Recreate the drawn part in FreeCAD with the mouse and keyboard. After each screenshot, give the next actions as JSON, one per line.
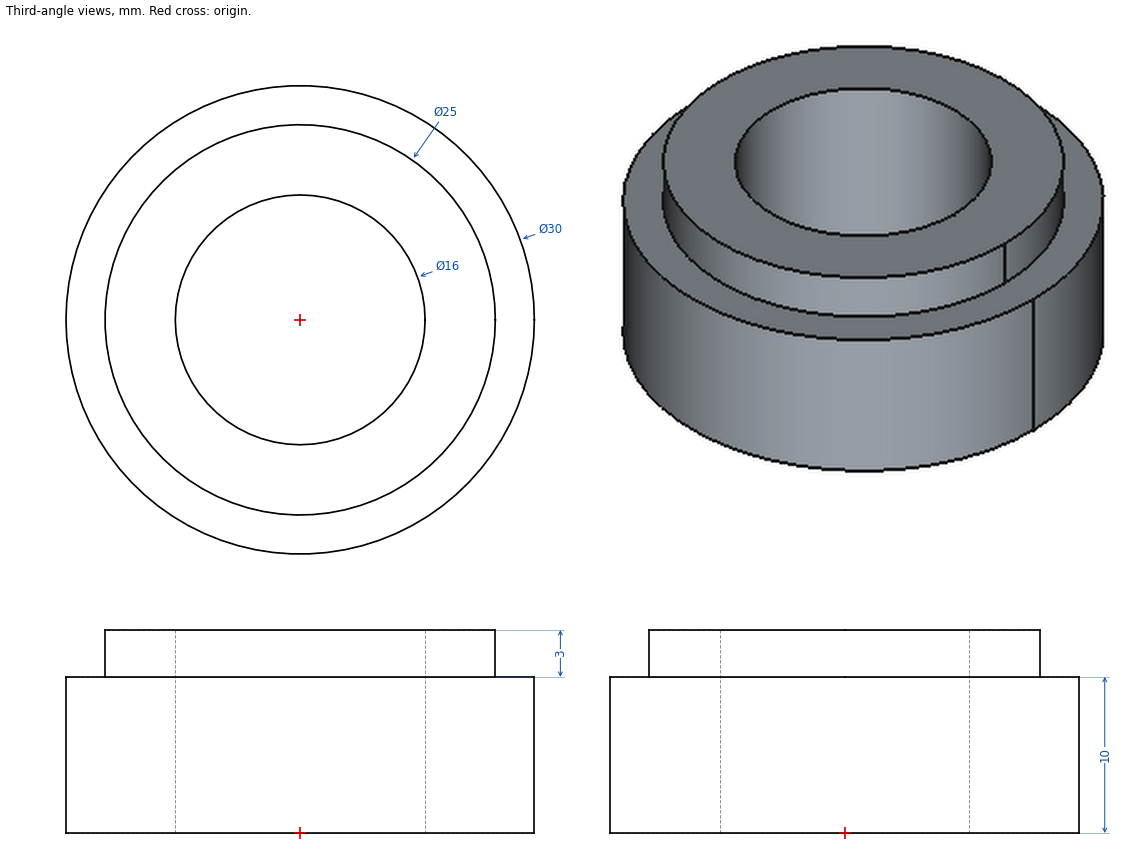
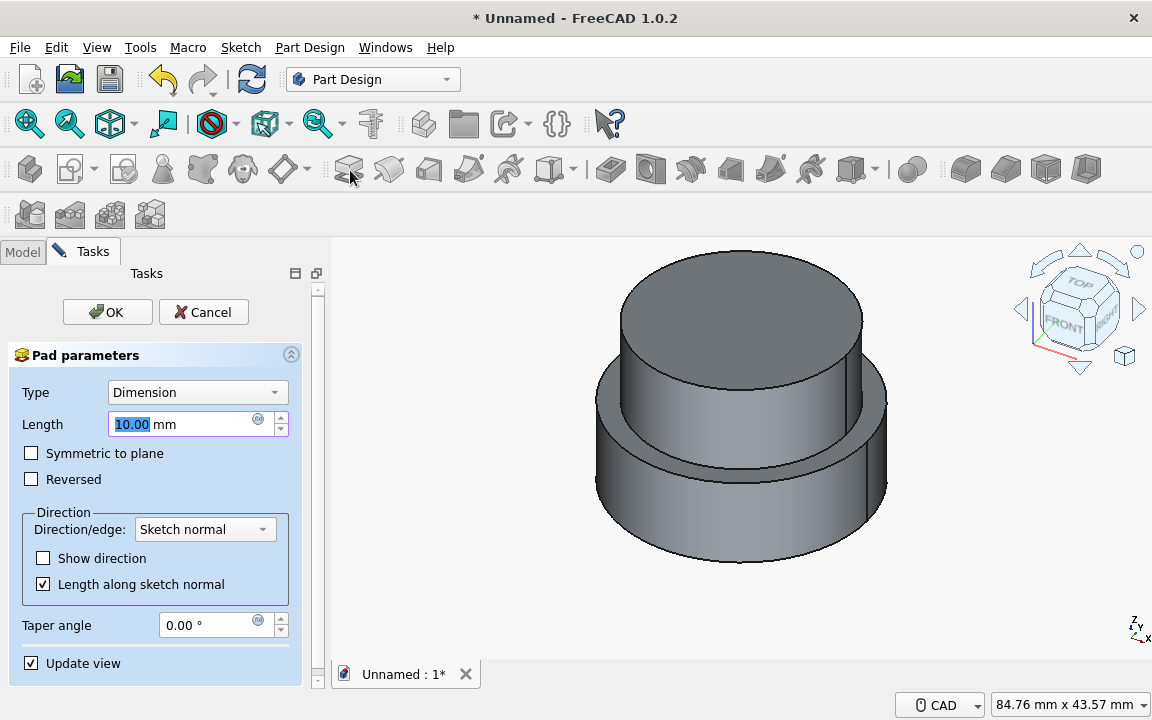
{"action": "type", "text": "3"}
{"action": "key", "text": "Tab"}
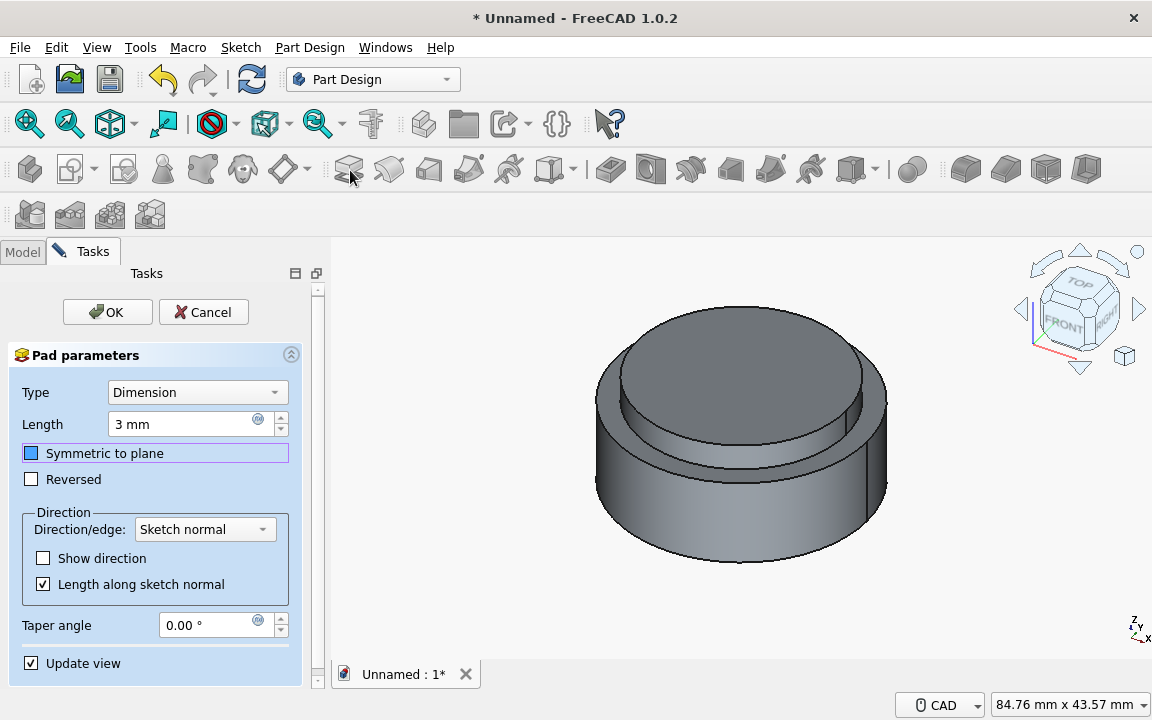
{"action": "left_click", "coordinate": [108, 312]}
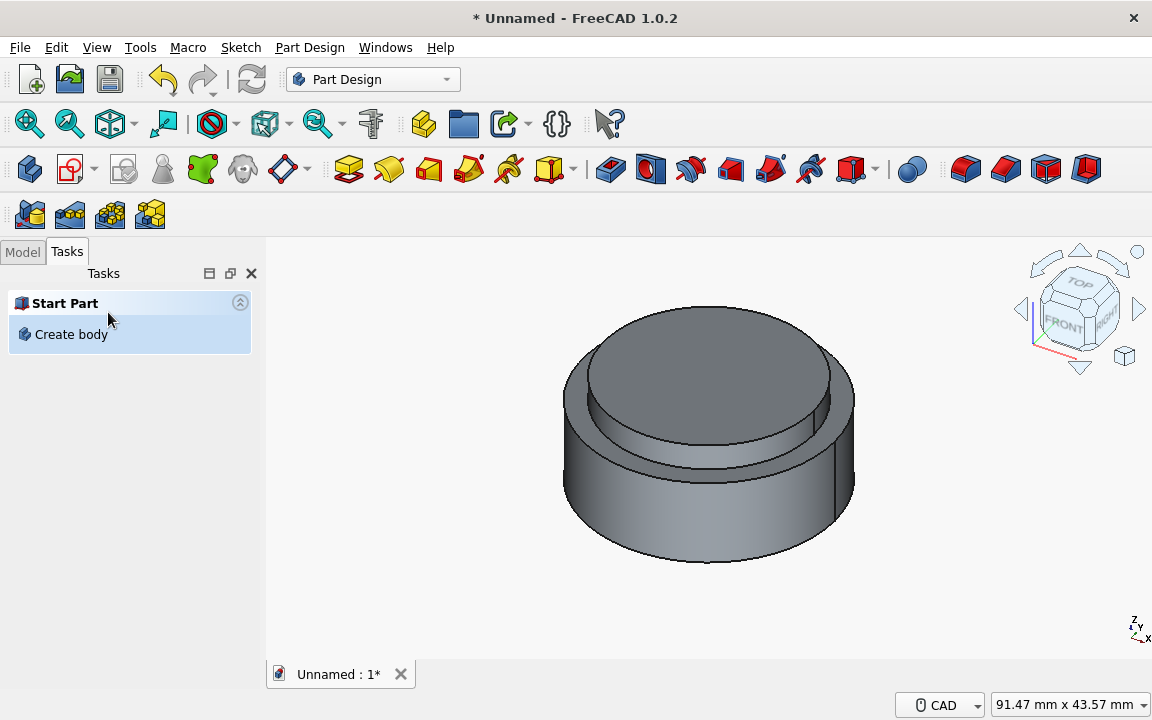
{"action": "left_click", "coordinate": [709, 375]}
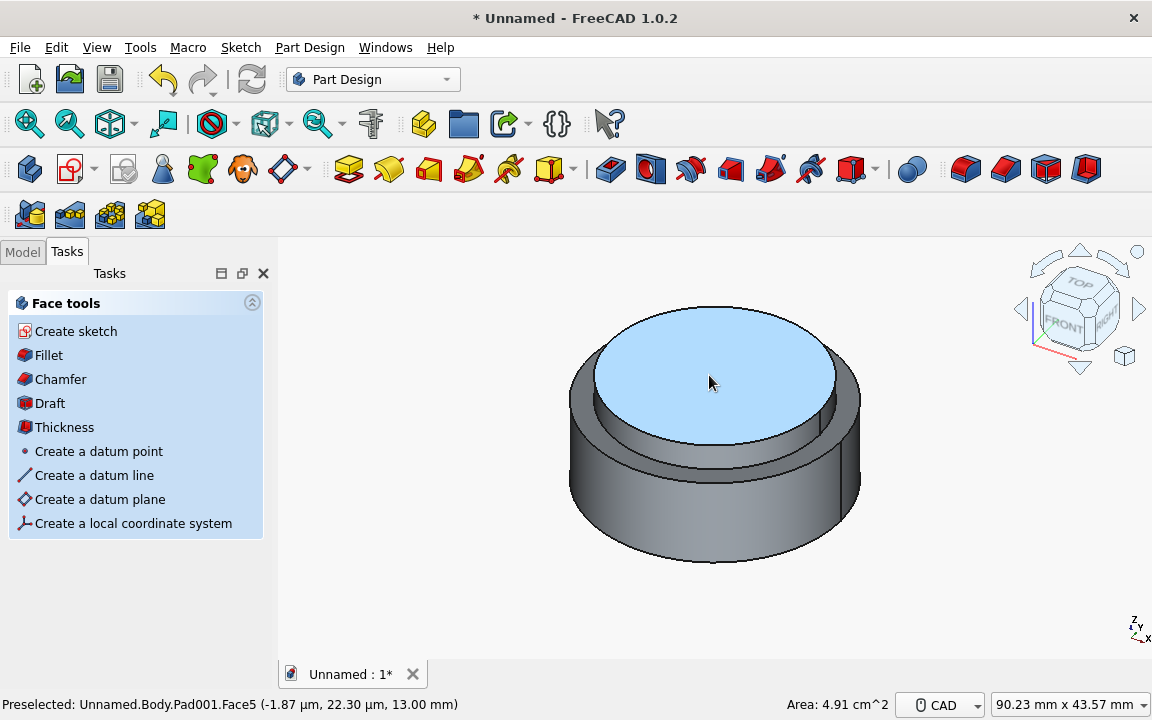
{"action": "left_click", "coordinate": [70, 170]}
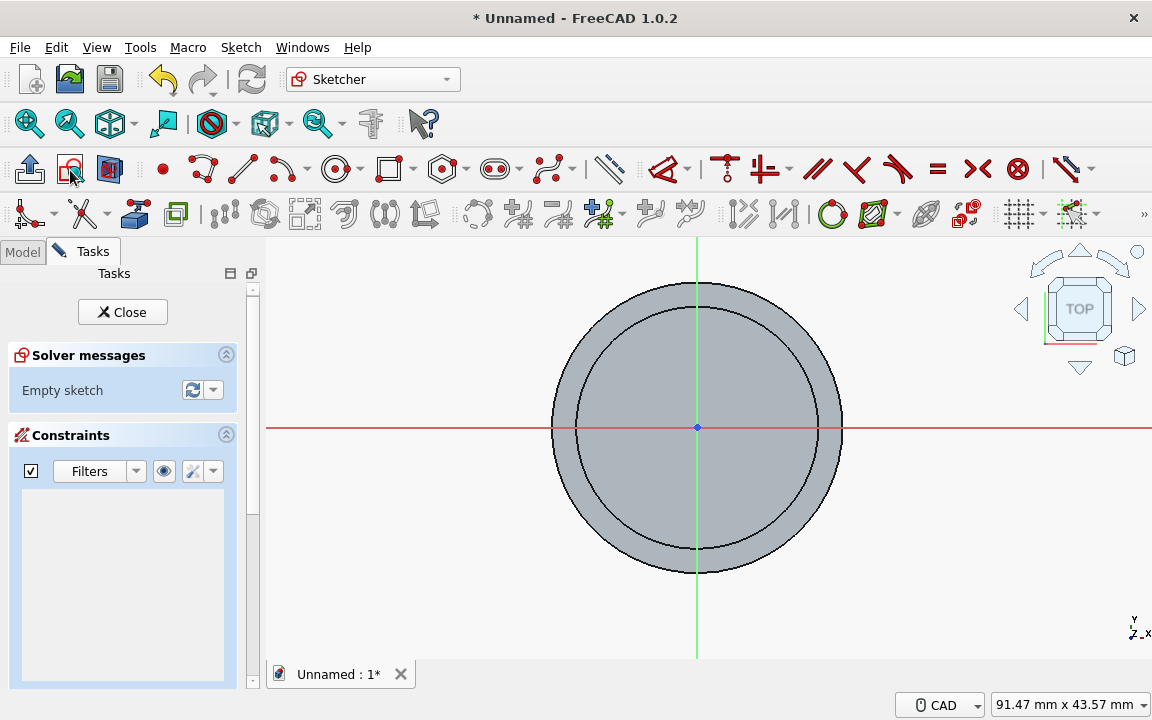
{"action": "scroll", "coordinate": [766, 403], "scroll_direction": "up", "scroll_amount": 3}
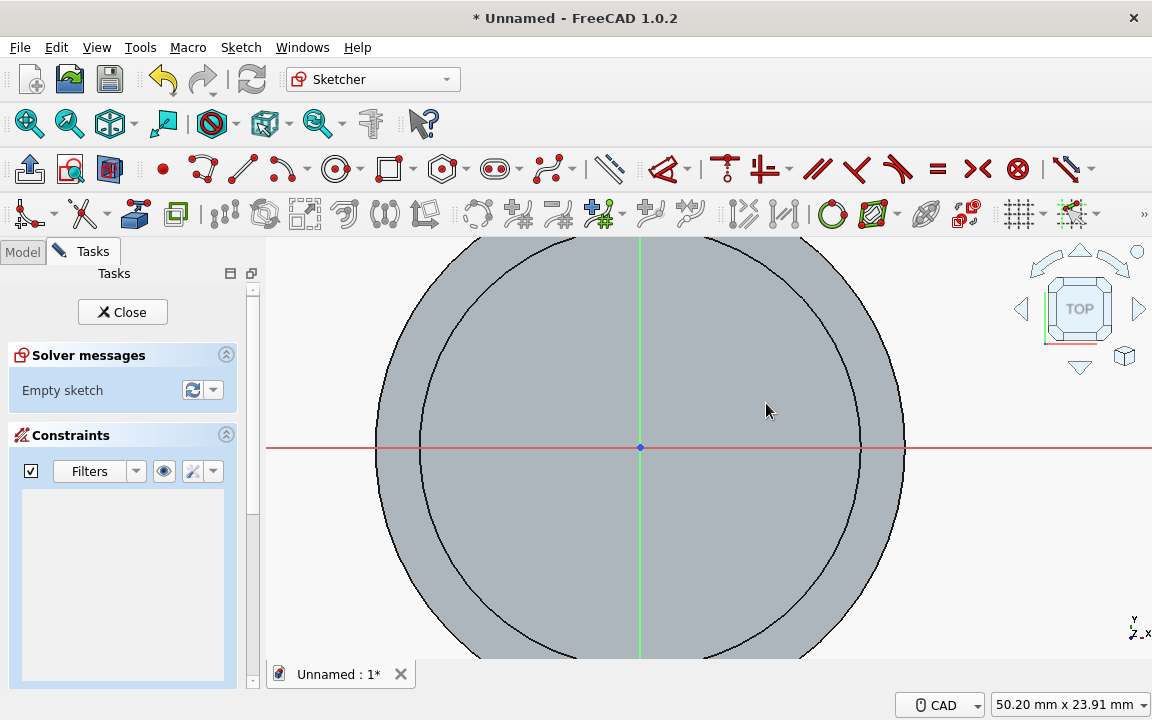
{"action": "key", "text": "g c"}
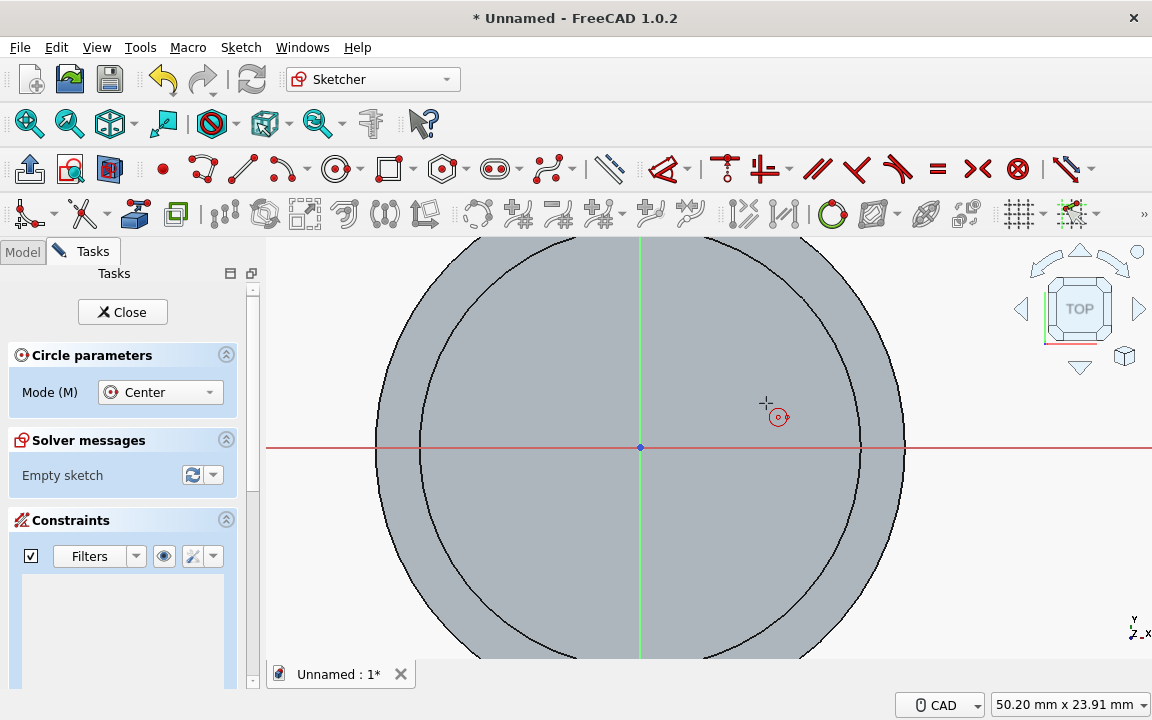
{"action": "left_click", "coordinate": [640, 448]}
{"action": "left_click", "coordinate": [740, 348]}
{"action": "key", "text": "Escape"}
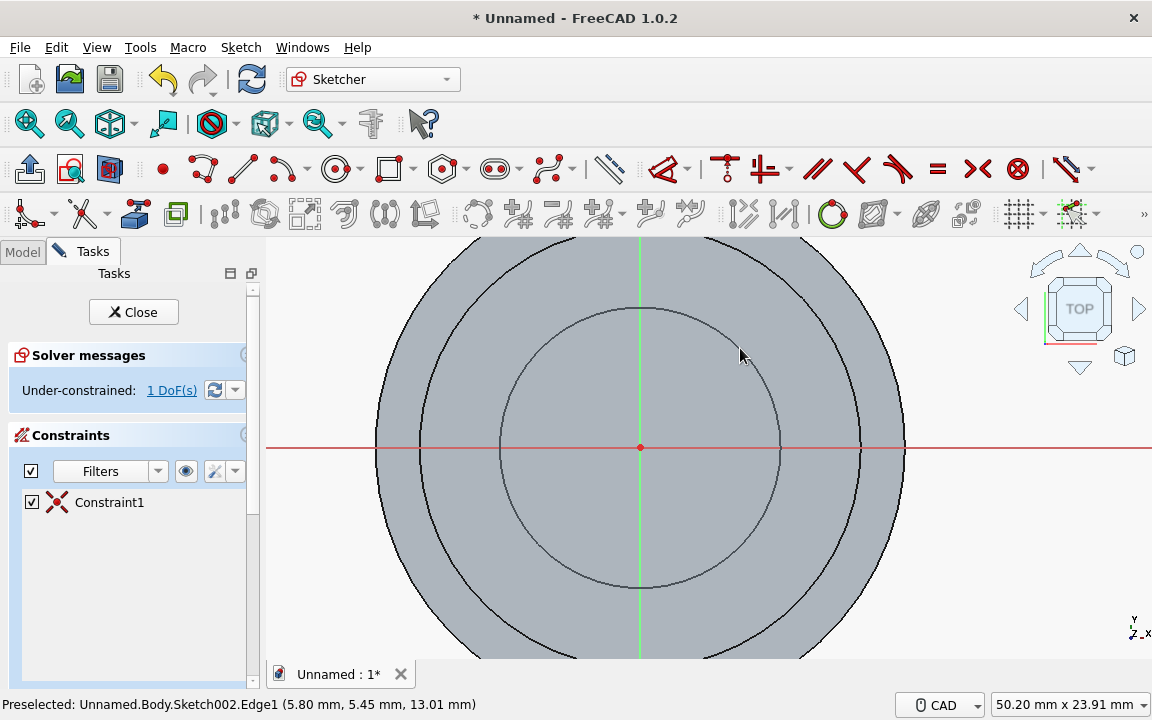
{"action": "left_click", "coordinate": [739, 348]}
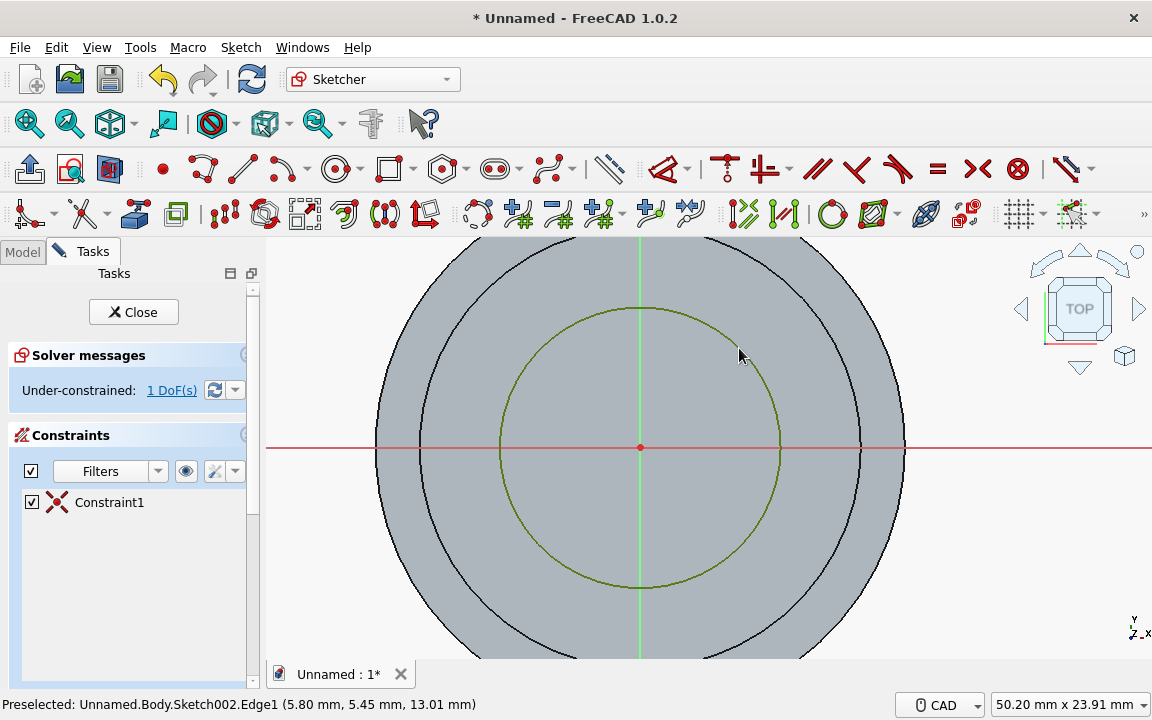
{"action": "left_click", "coordinate": [690, 170]}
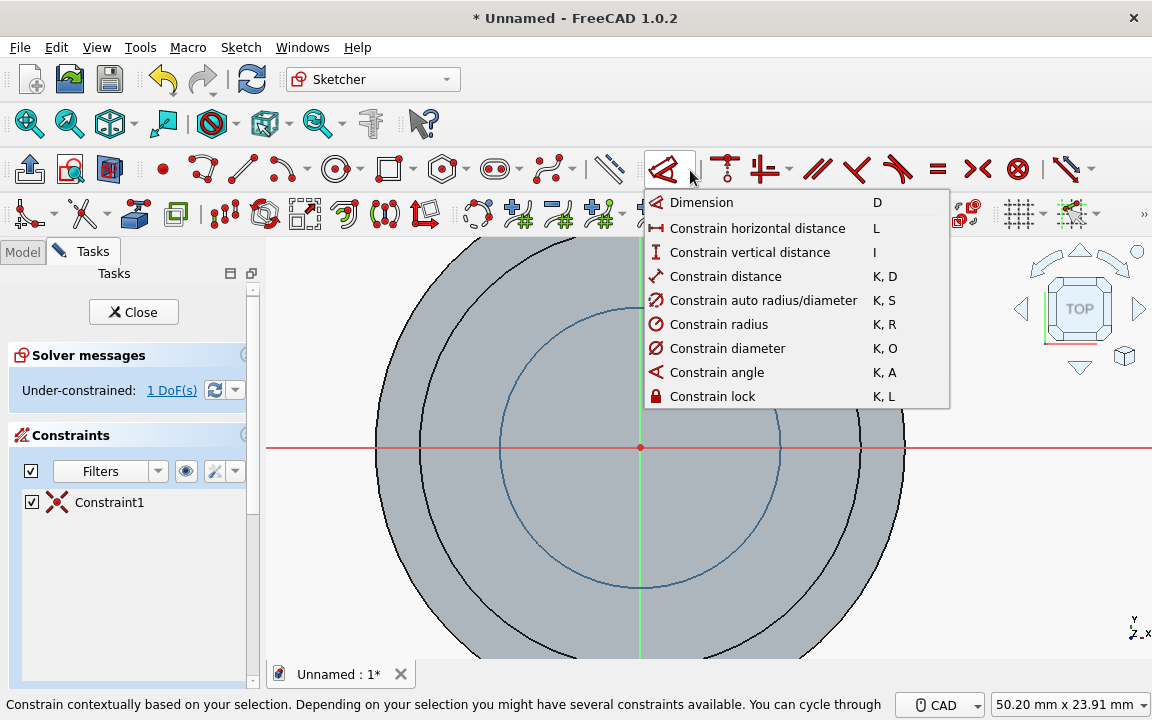
{"action": "left_click", "coordinate": [797, 348]}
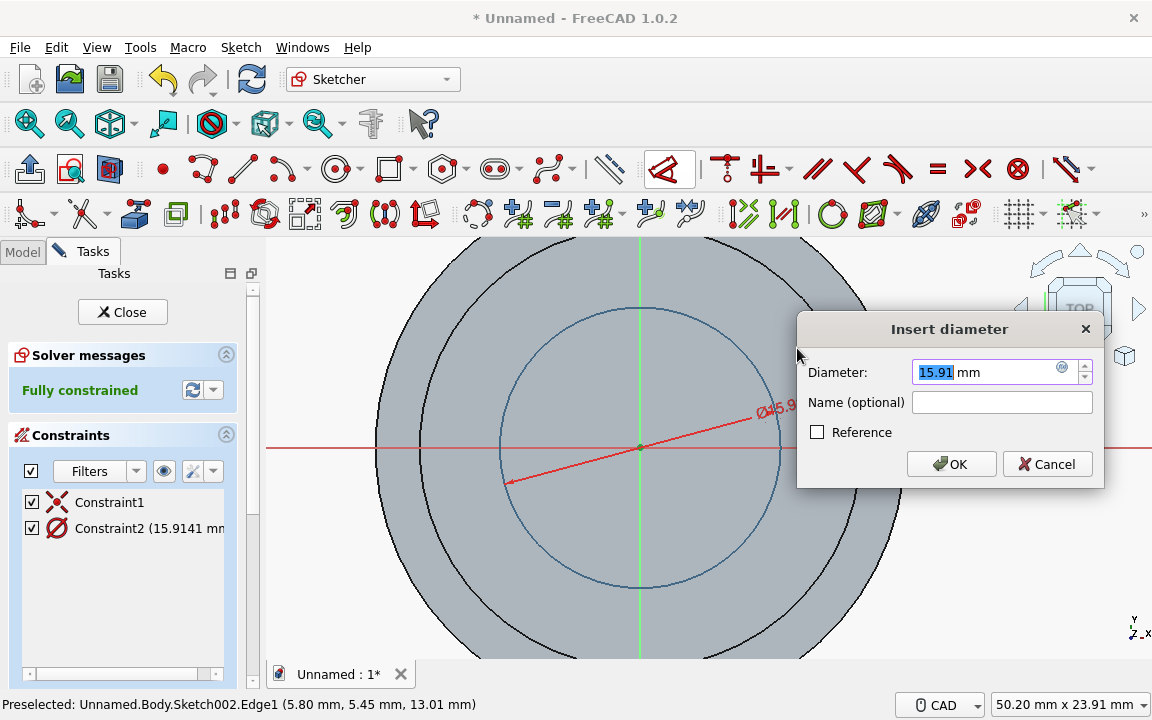
{"action": "type", "text": "16"}
{"action": "key", "text": "Return"}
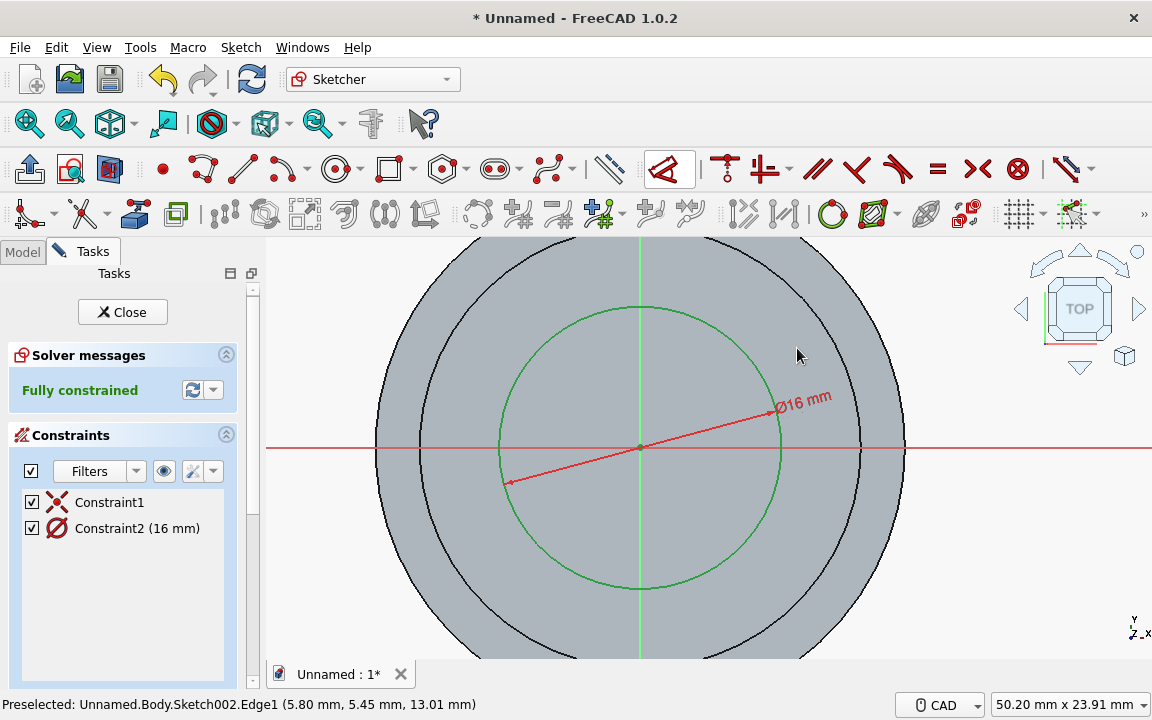
{"action": "left_click", "coordinate": [123, 312]}